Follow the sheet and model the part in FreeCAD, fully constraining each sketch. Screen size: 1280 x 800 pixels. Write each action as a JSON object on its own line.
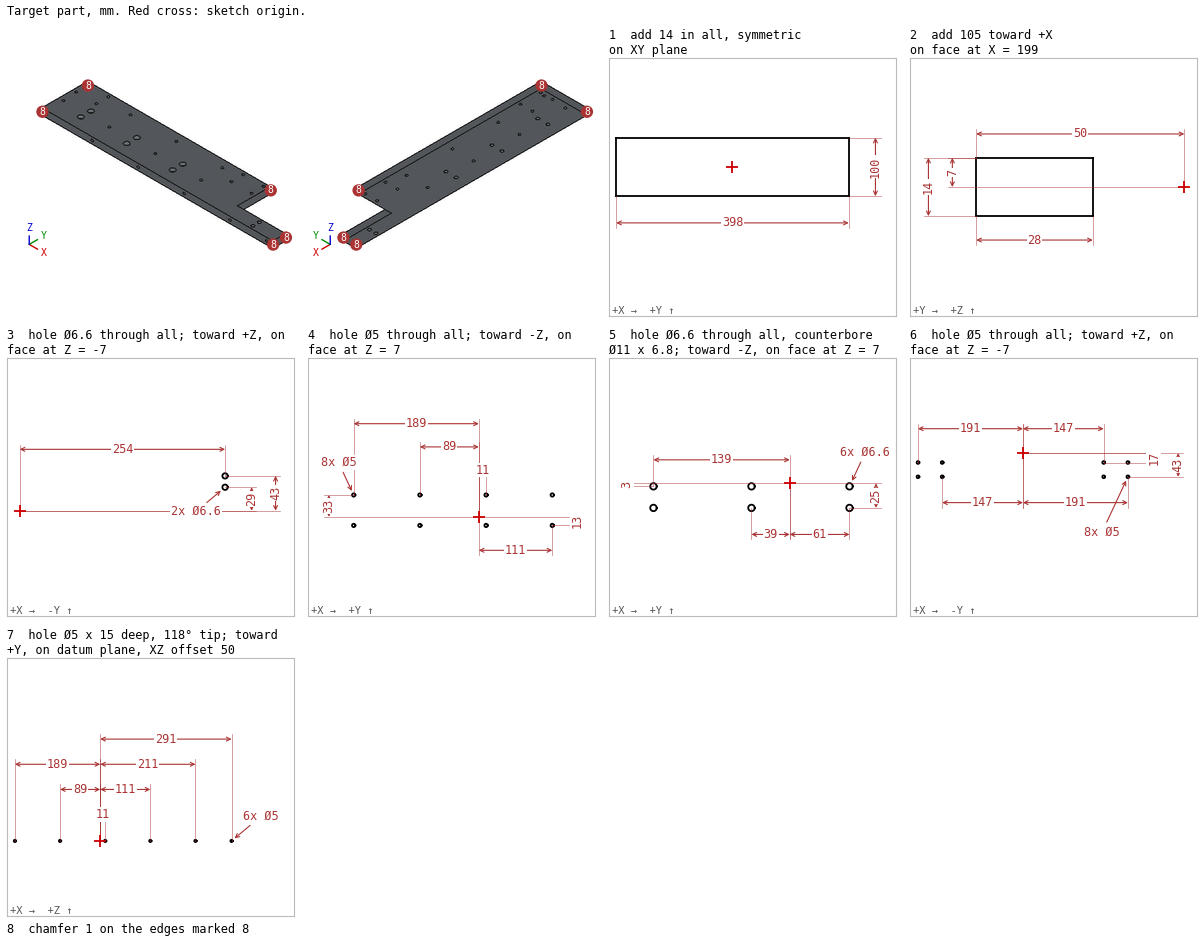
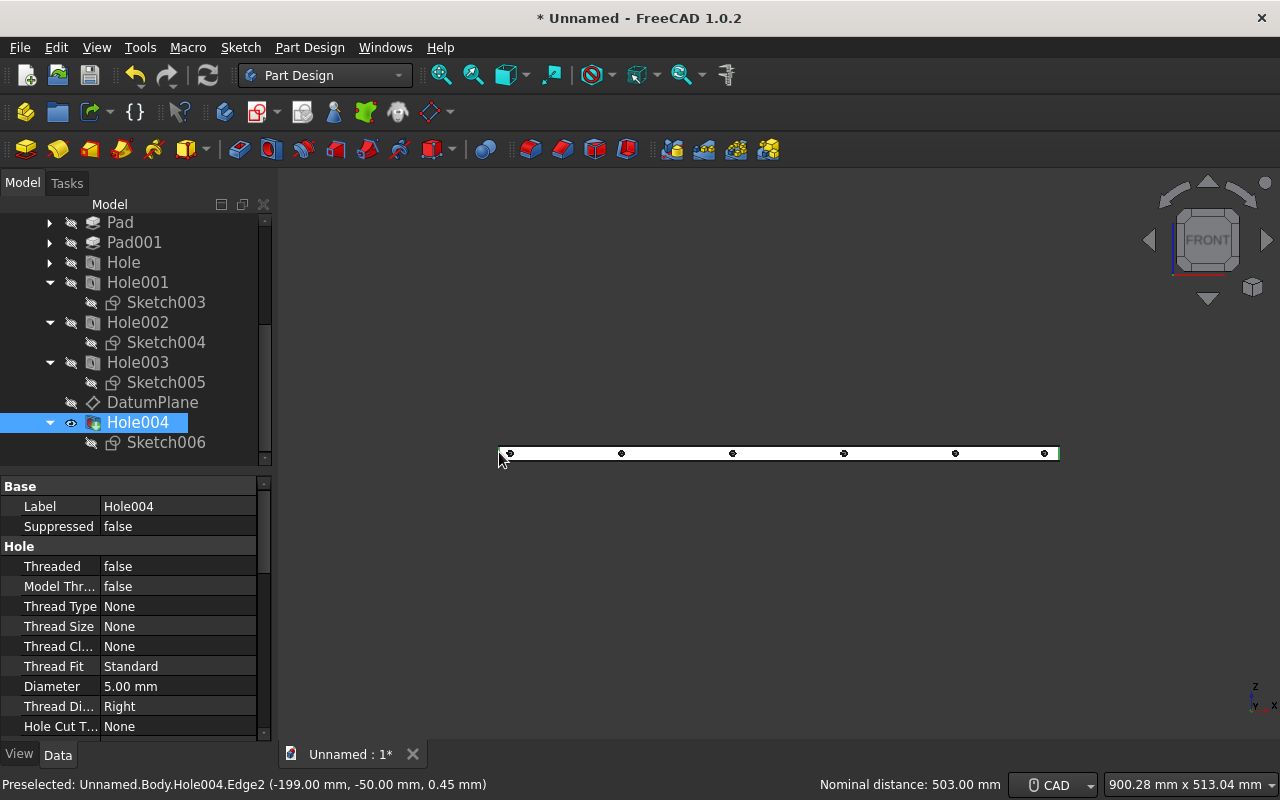
{"action": "scroll", "coordinate": [1059, 452], "scroll_direction": "up", "scroll_amount": 5}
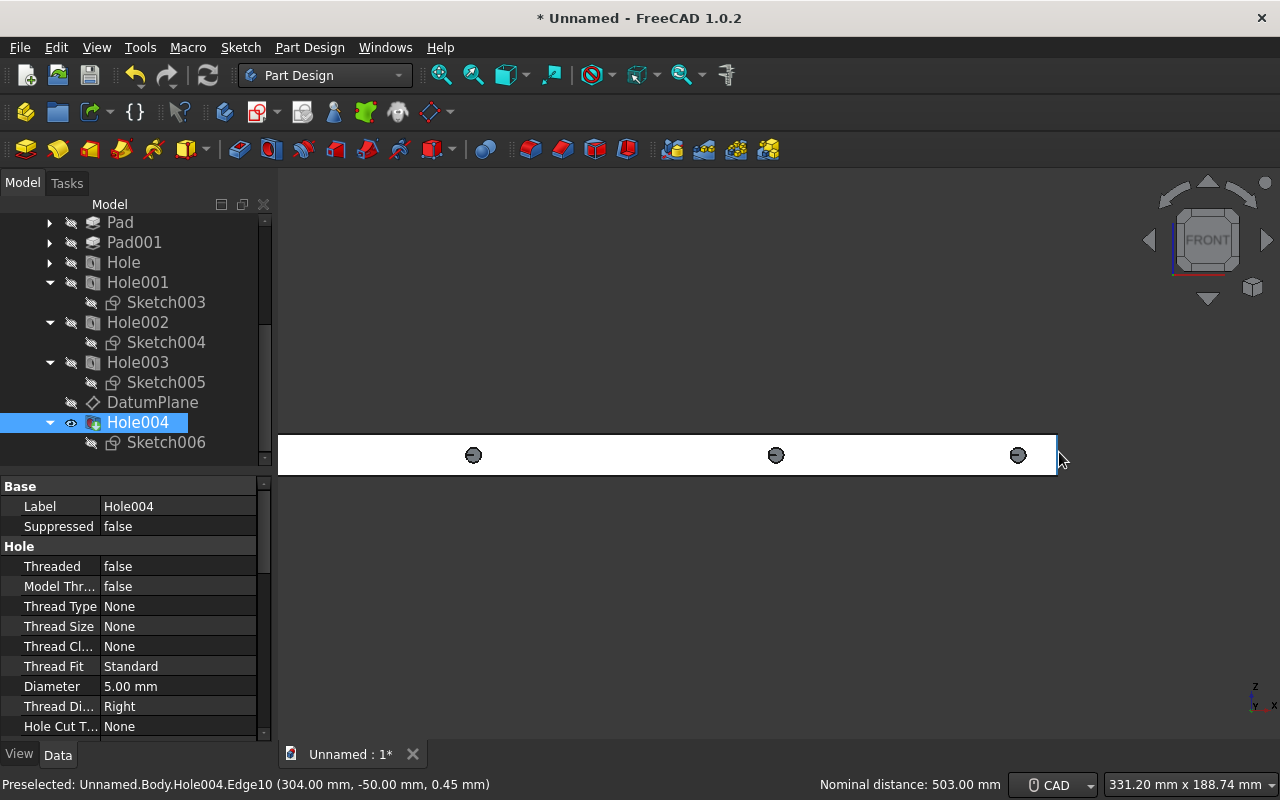
{"action": "left_click", "coordinate": [442, 76]}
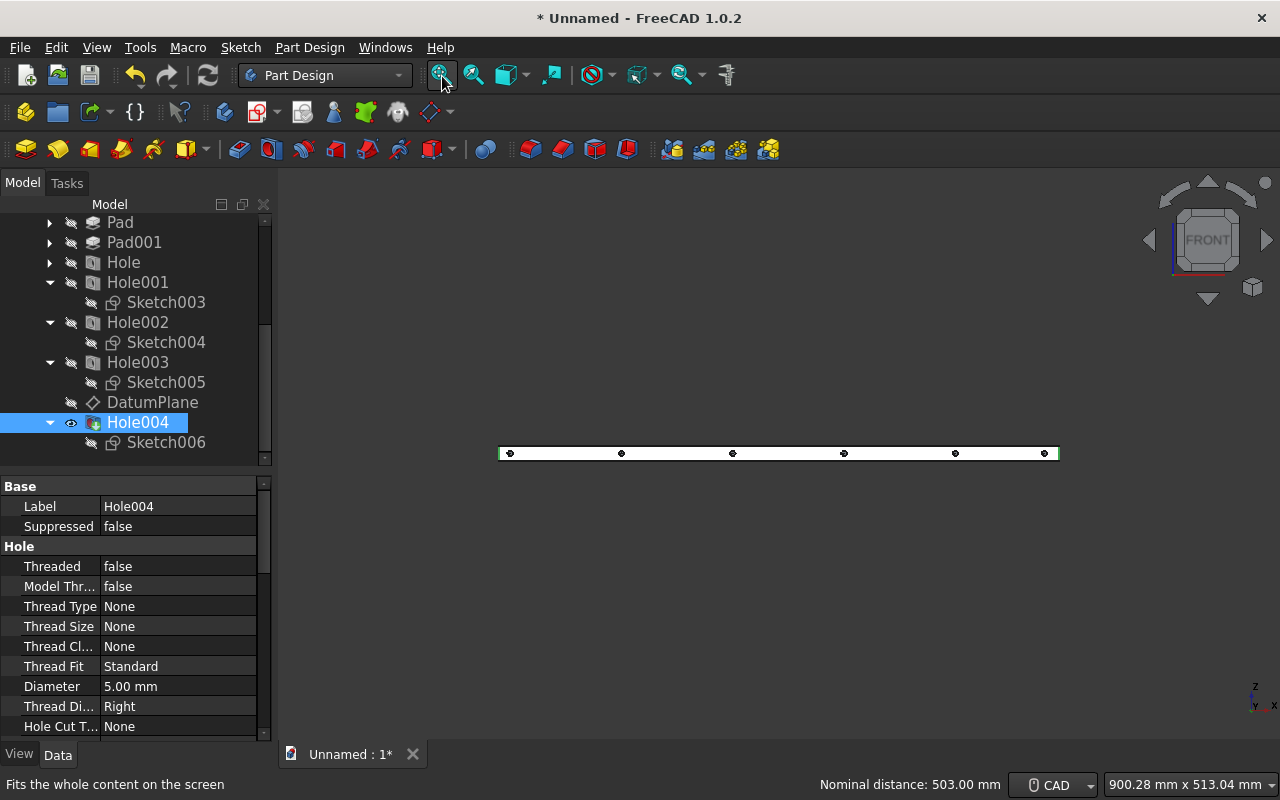
{"action": "key", "text": "3"}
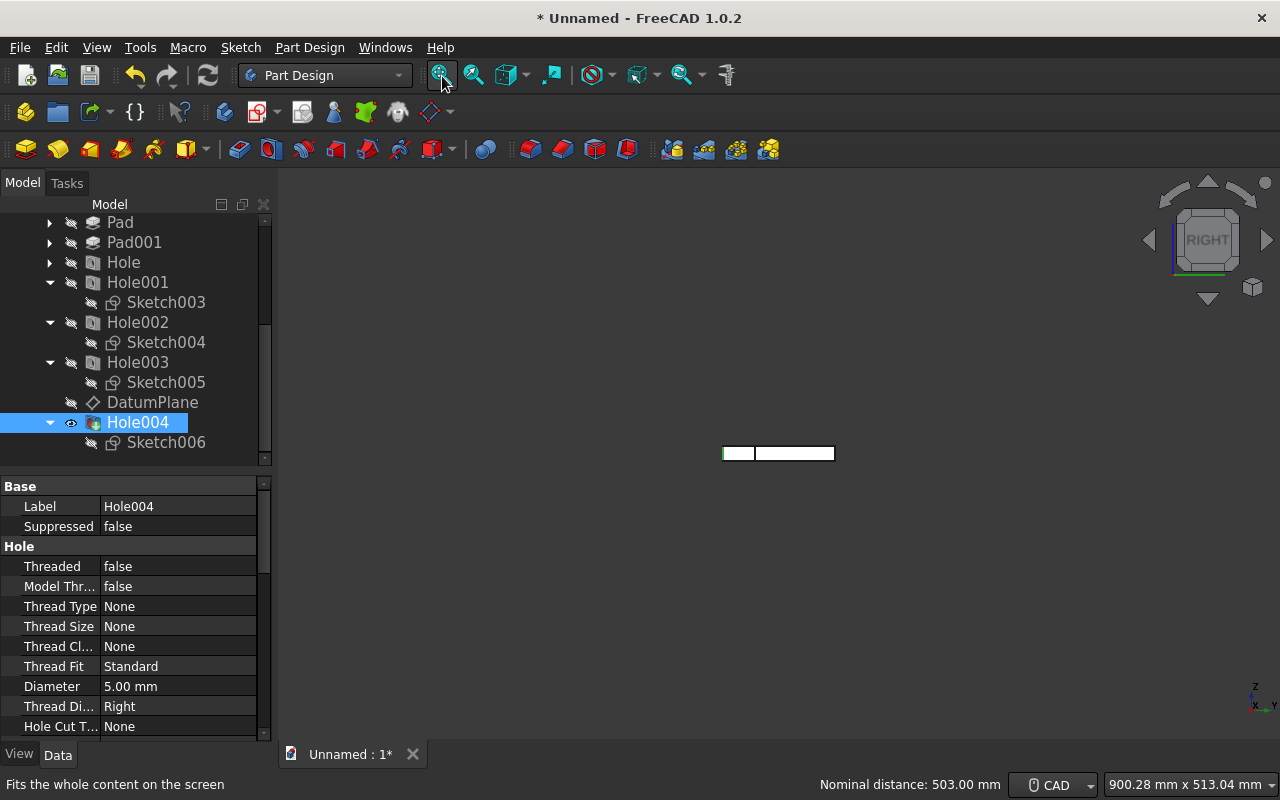
{"action": "key", "text": "v f"}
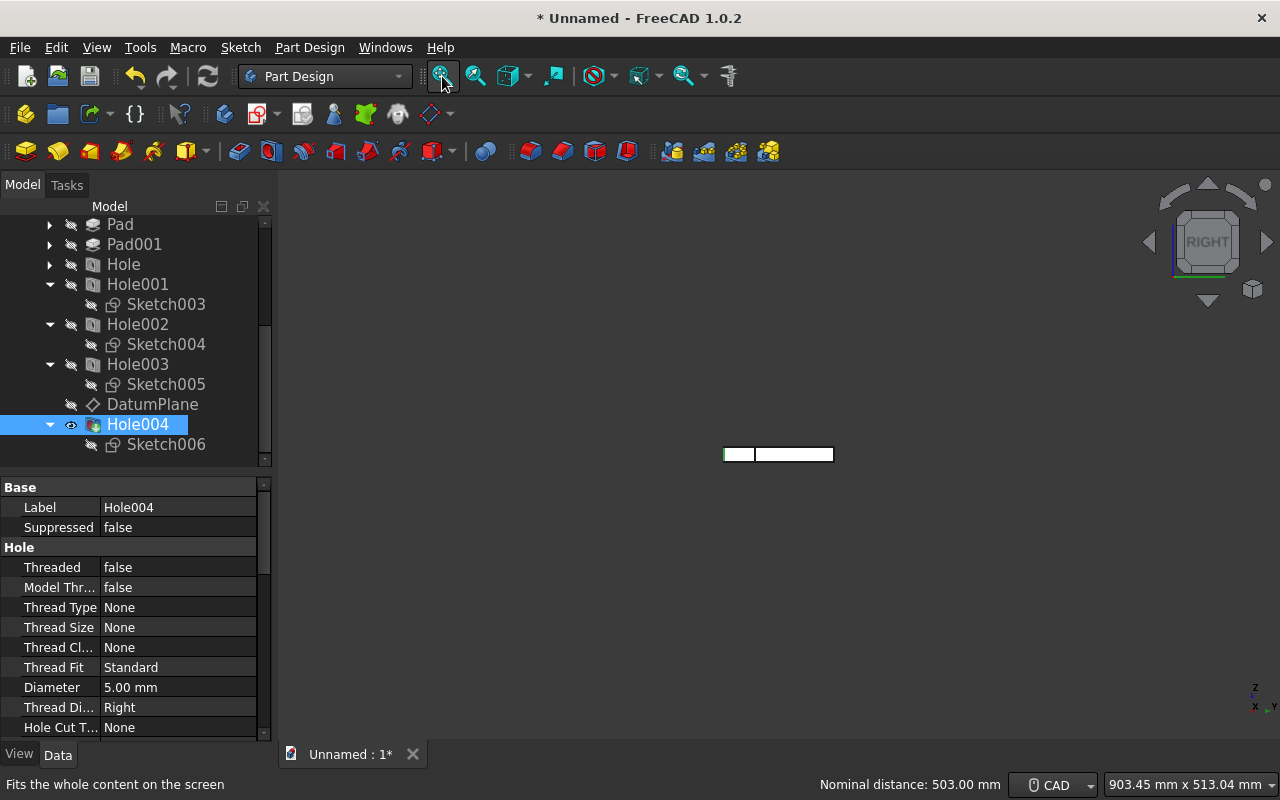
{"action": "left_click", "coordinate": [755, 453], "text": "ctrl"}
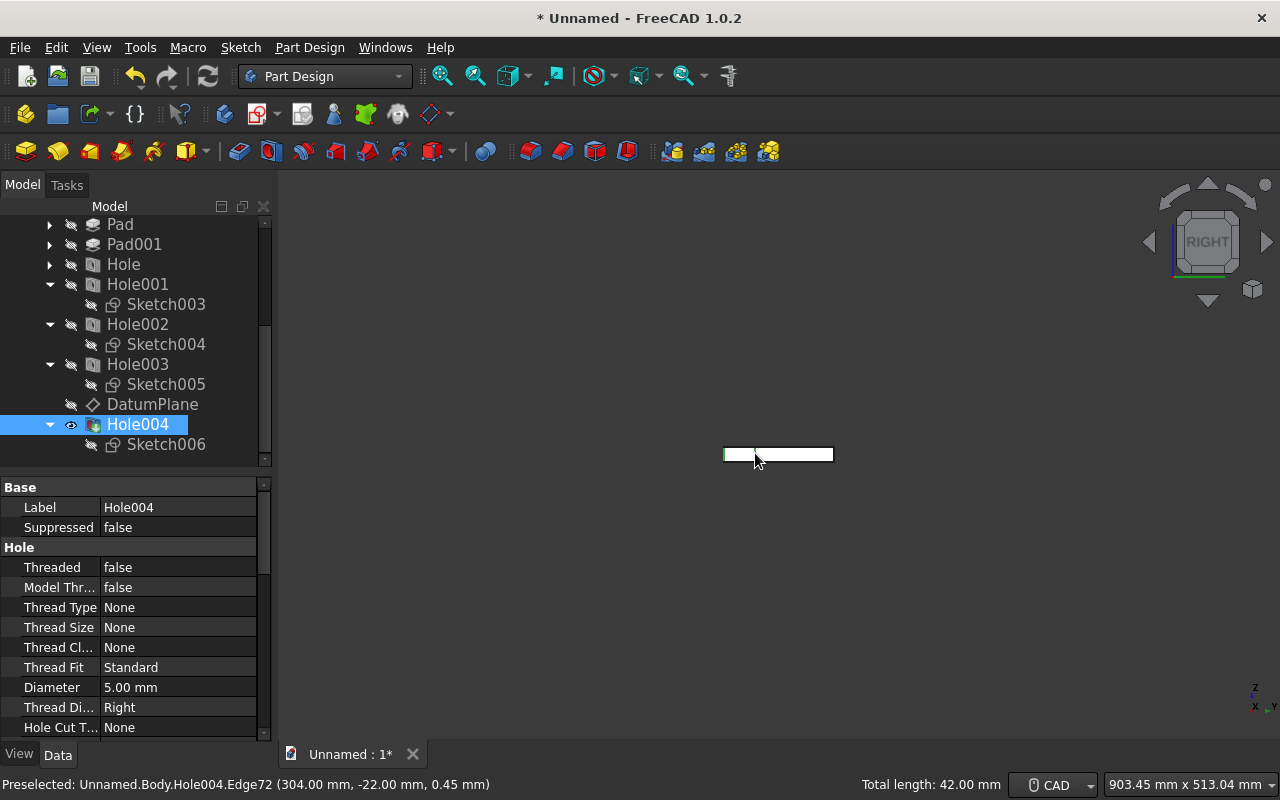
{"action": "left_click", "coordinate": [834, 453], "text": "ctrl"}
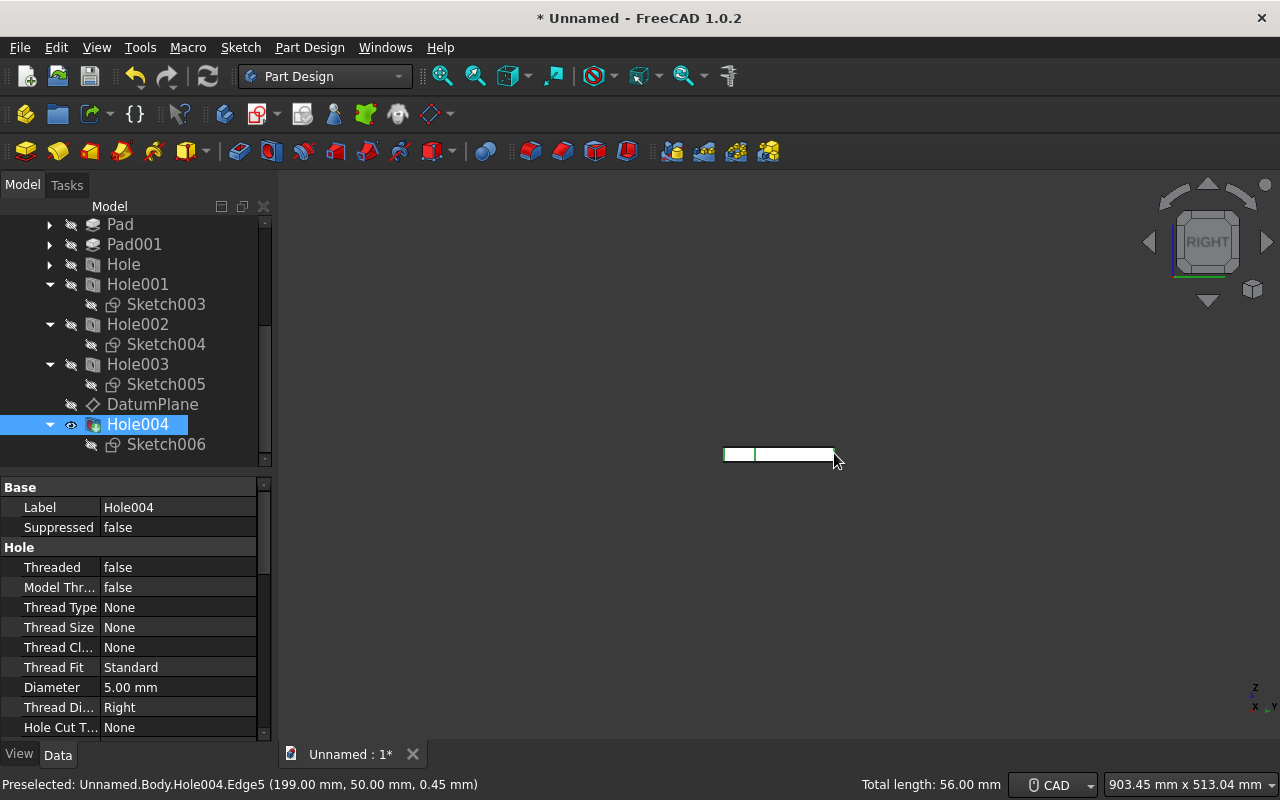
{"action": "scroll", "coordinate": [834, 453], "scroll_direction": "up", "scroll_amount": 5}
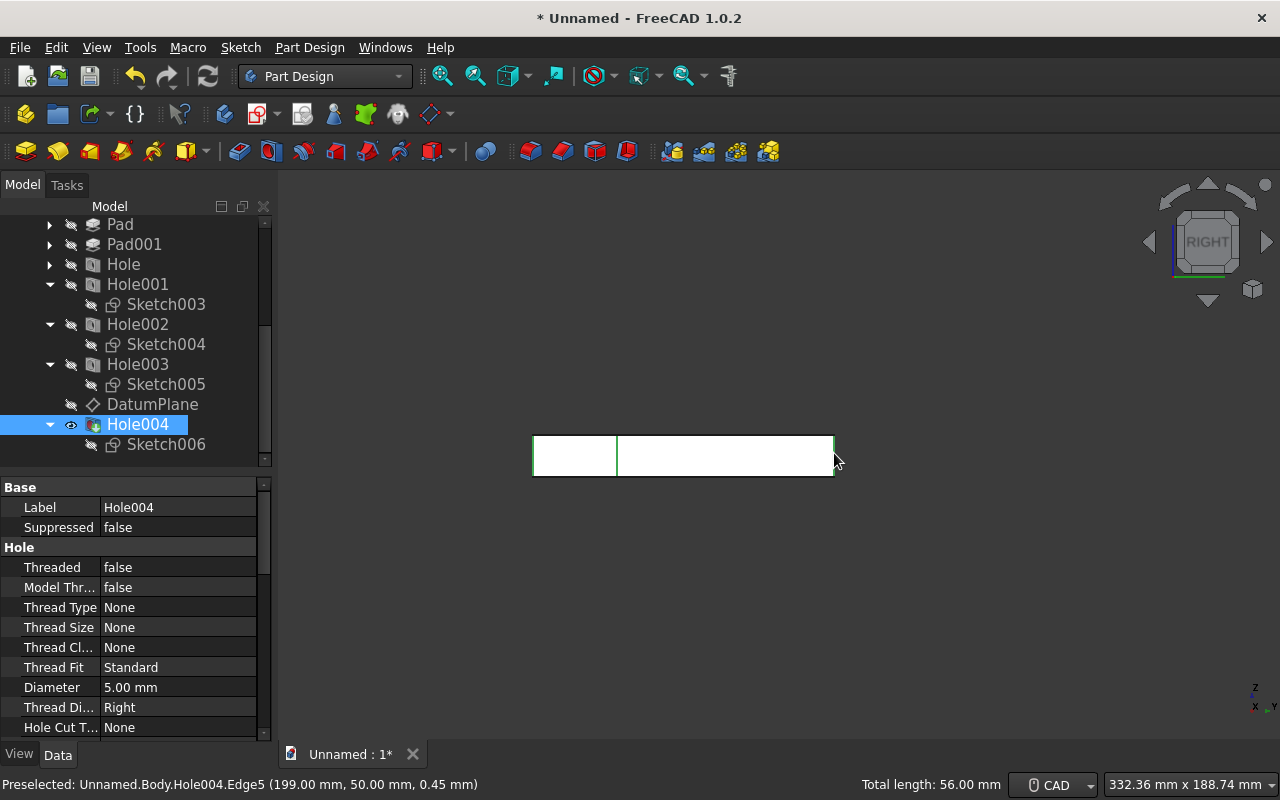
{"action": "left_click", "coordinate": [444, 76]}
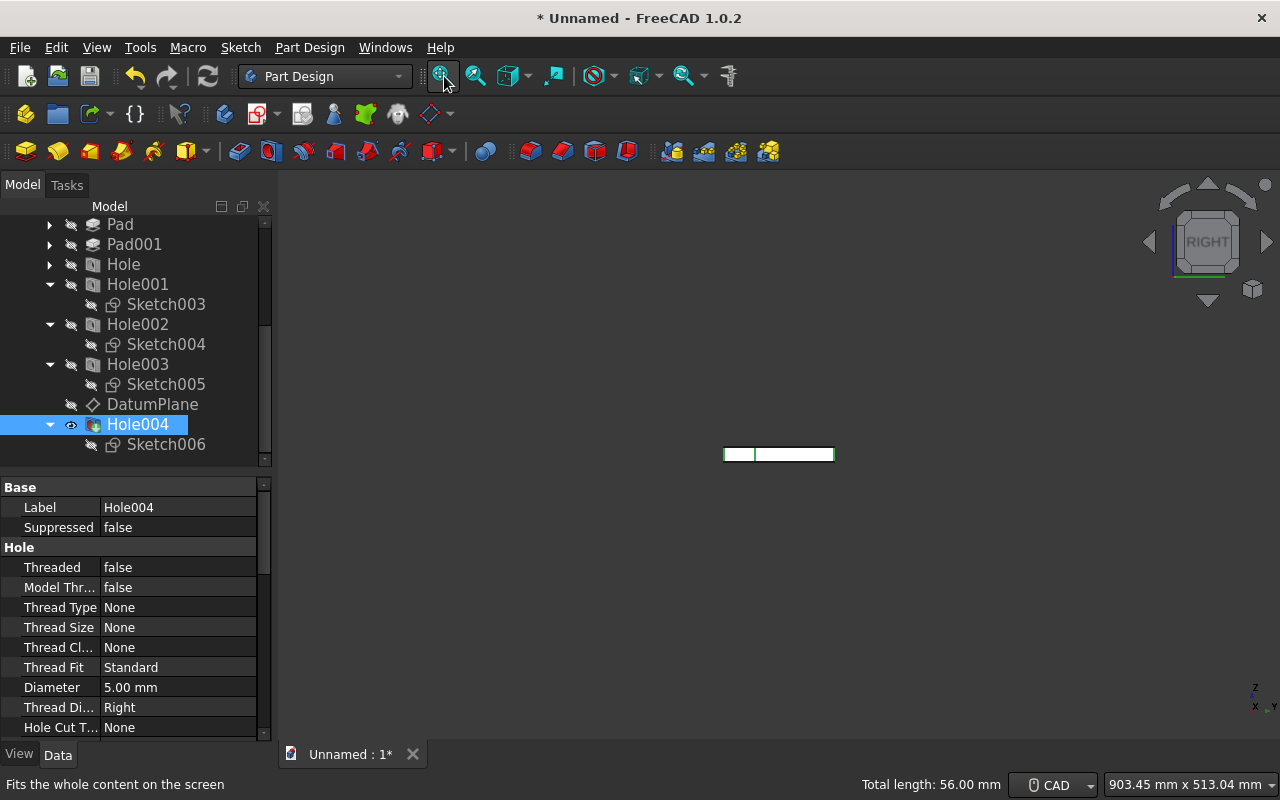
{"action": "key", "text": "5"}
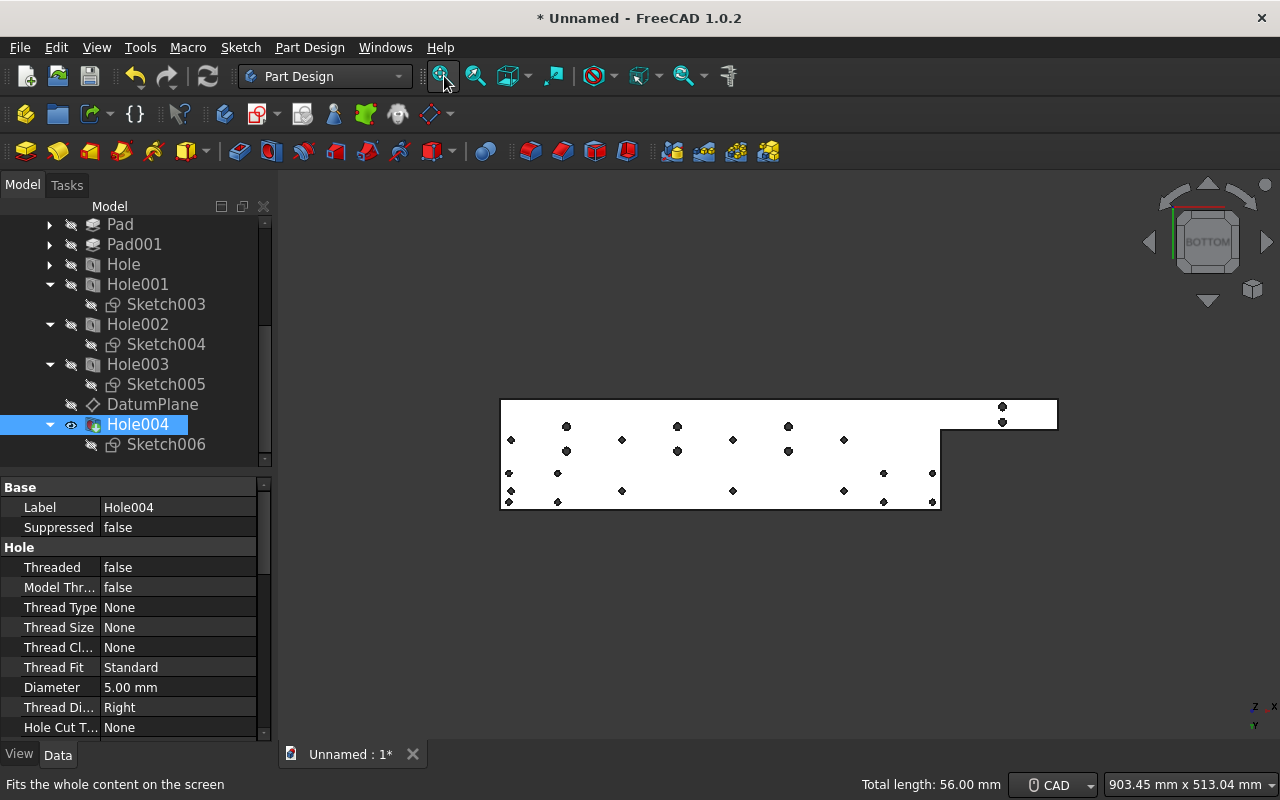
{"action": "scroll", "coordinate": [500, 509], "scroll_direction": "up", "scroll_amount": 5}